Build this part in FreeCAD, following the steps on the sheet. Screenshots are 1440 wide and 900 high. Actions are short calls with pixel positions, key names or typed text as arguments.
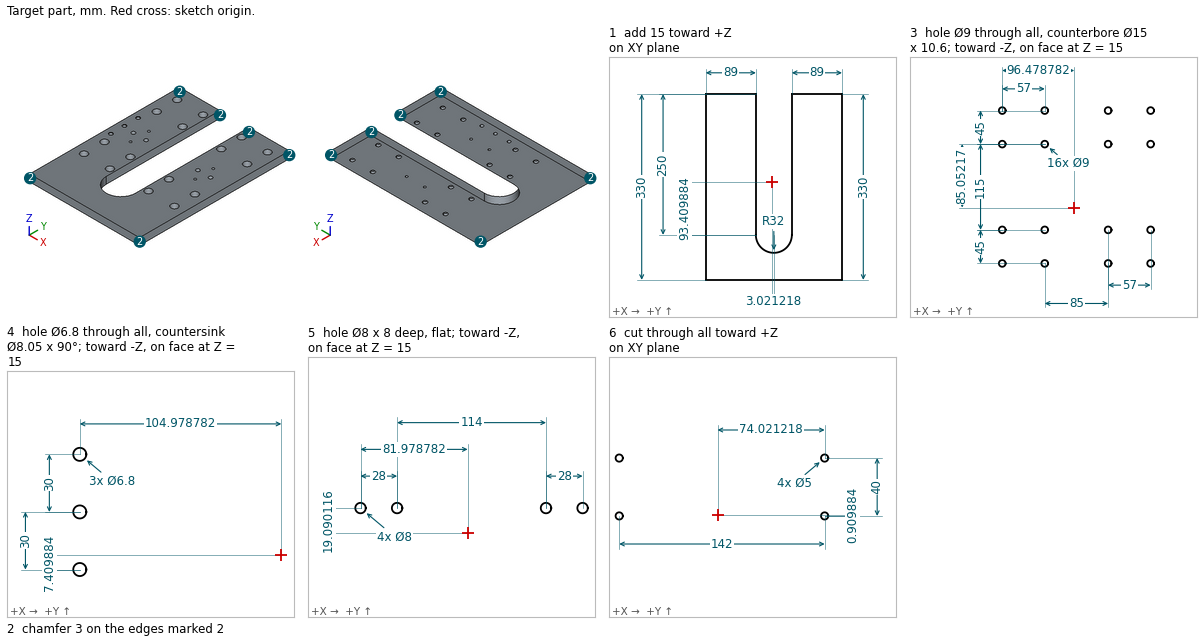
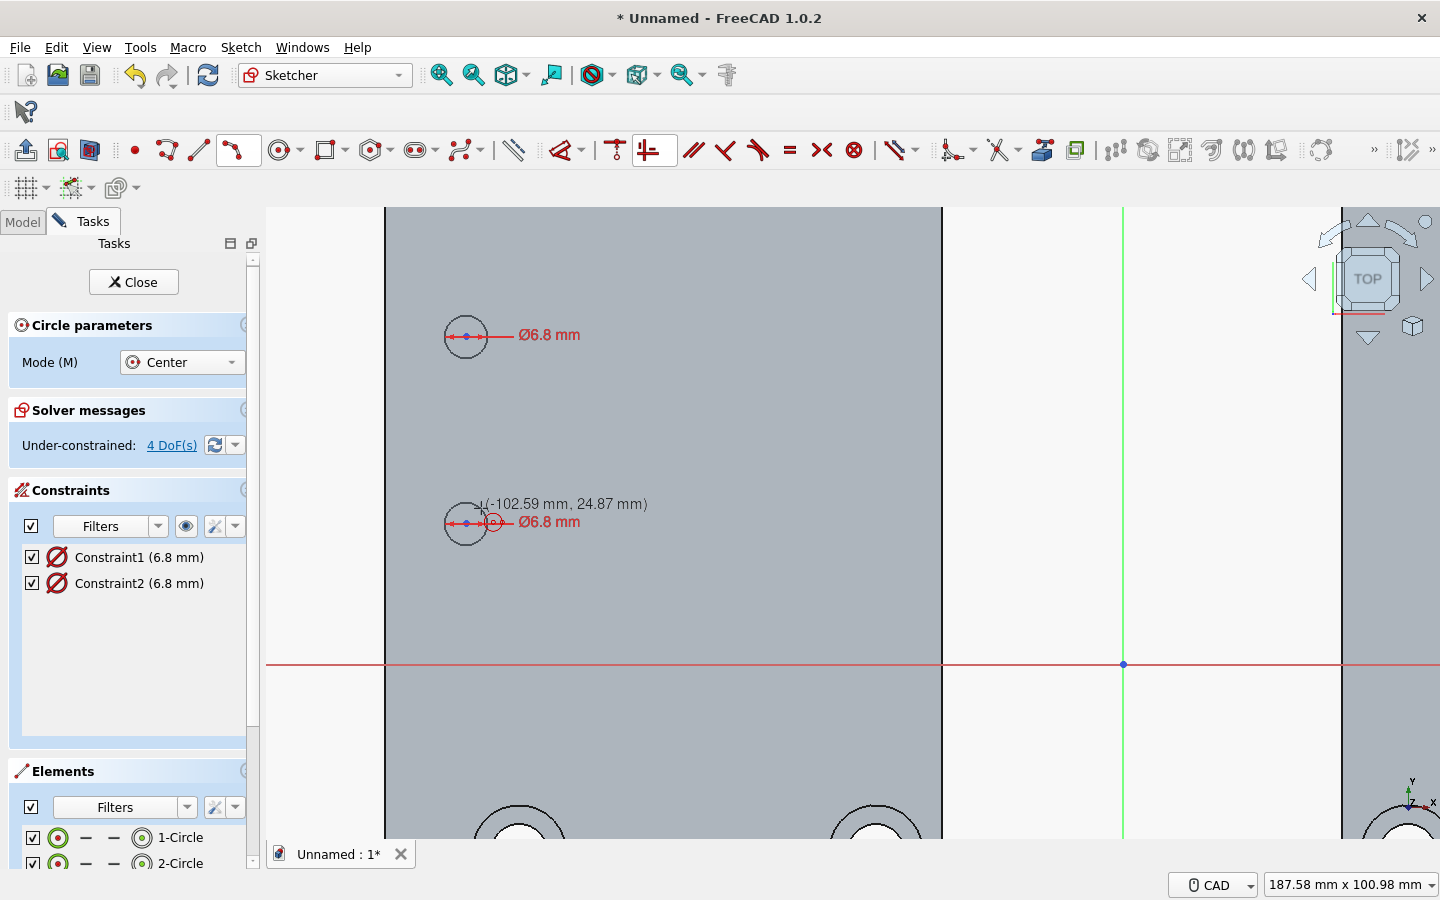
click(466, 711)
move(481, 696)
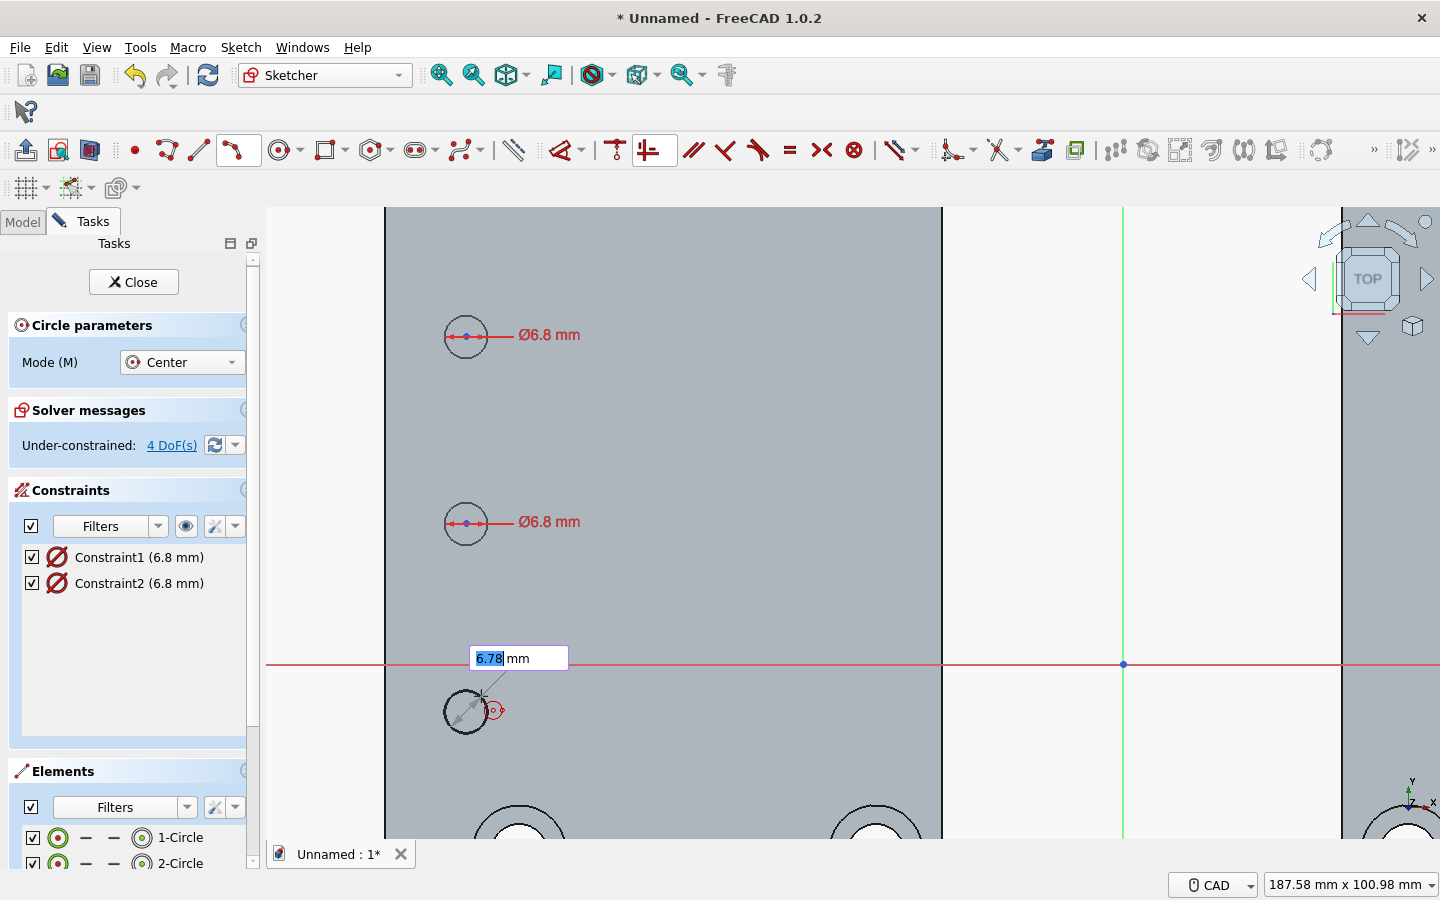
text(6.8)
key(Return)
key(Escape)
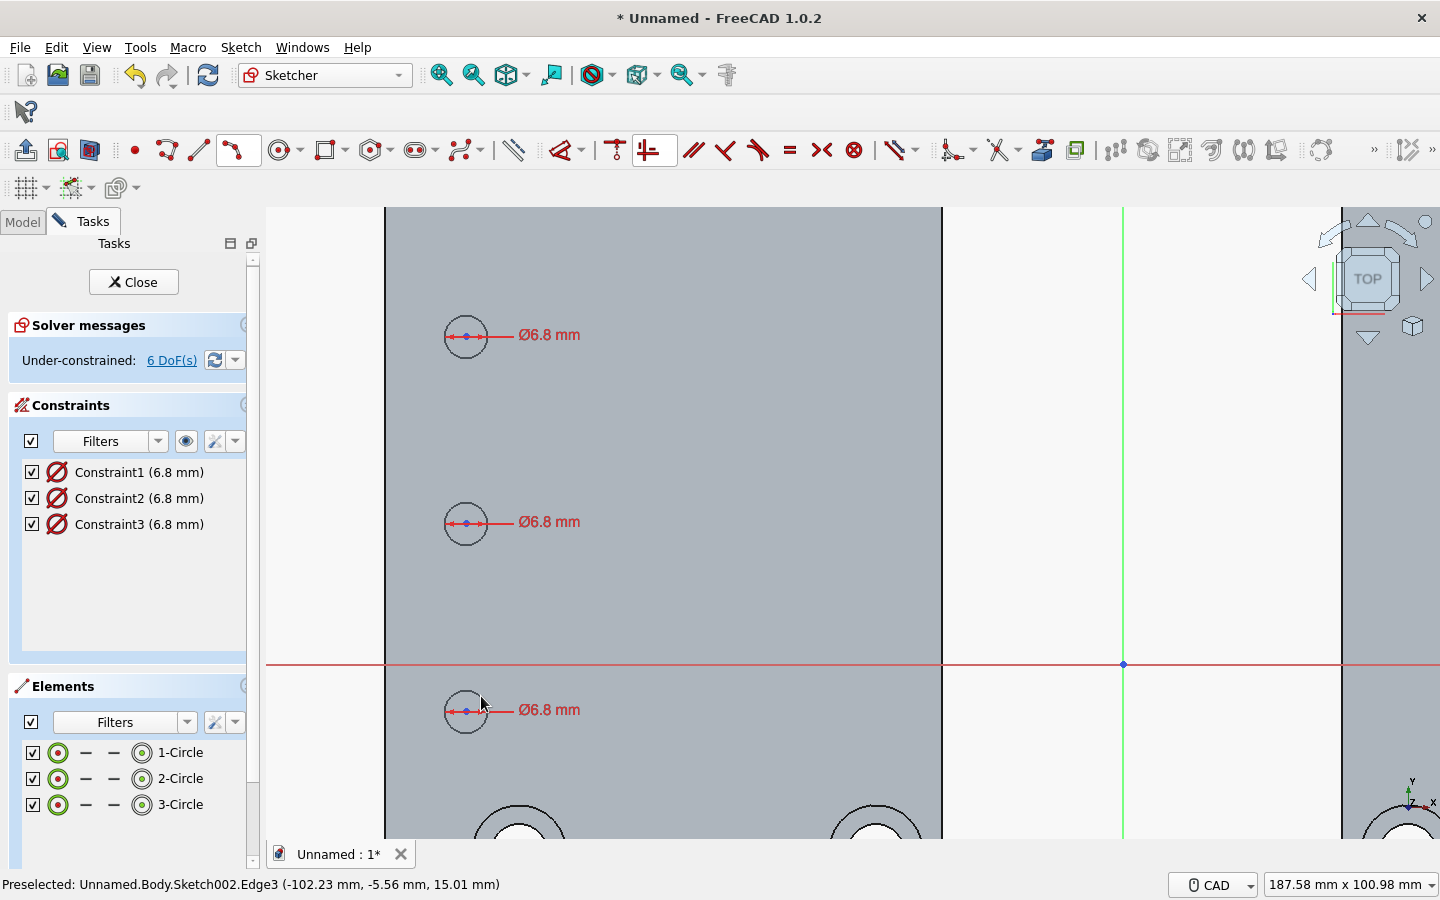
click(466, 337)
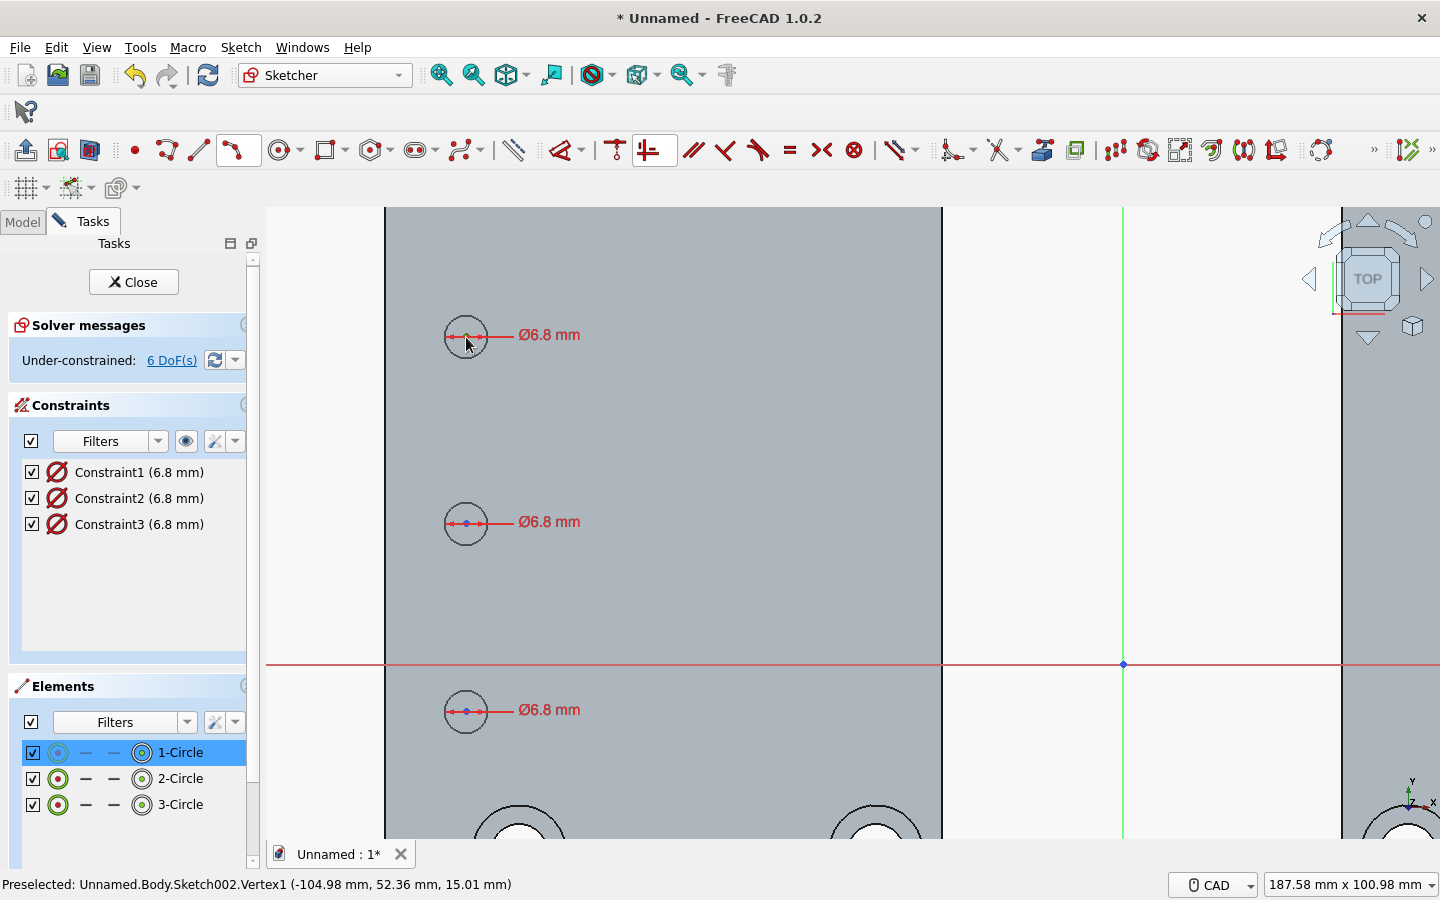
click(466, 524)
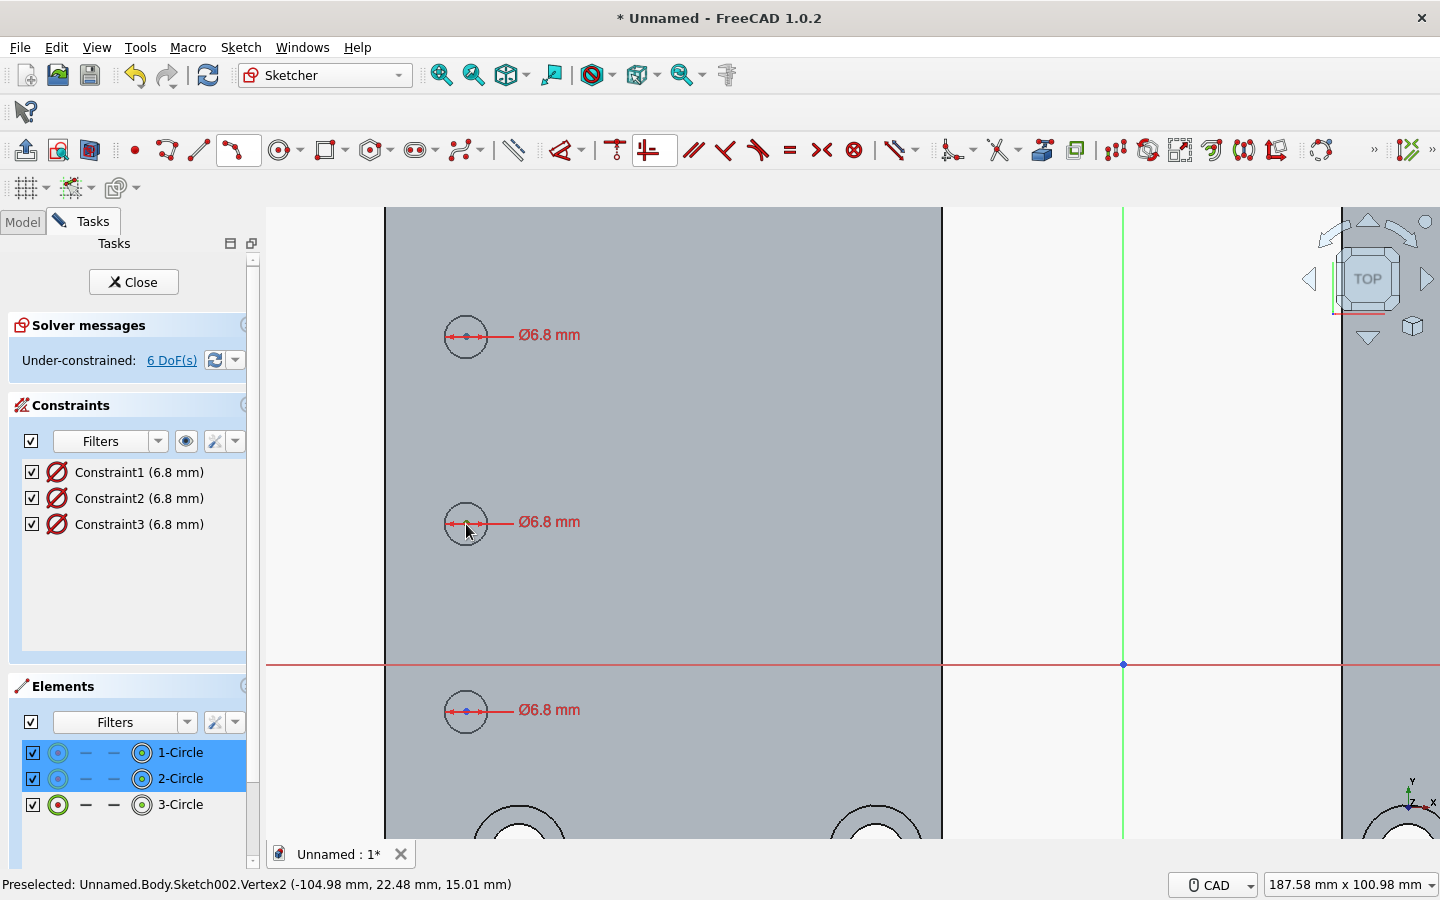
key(v)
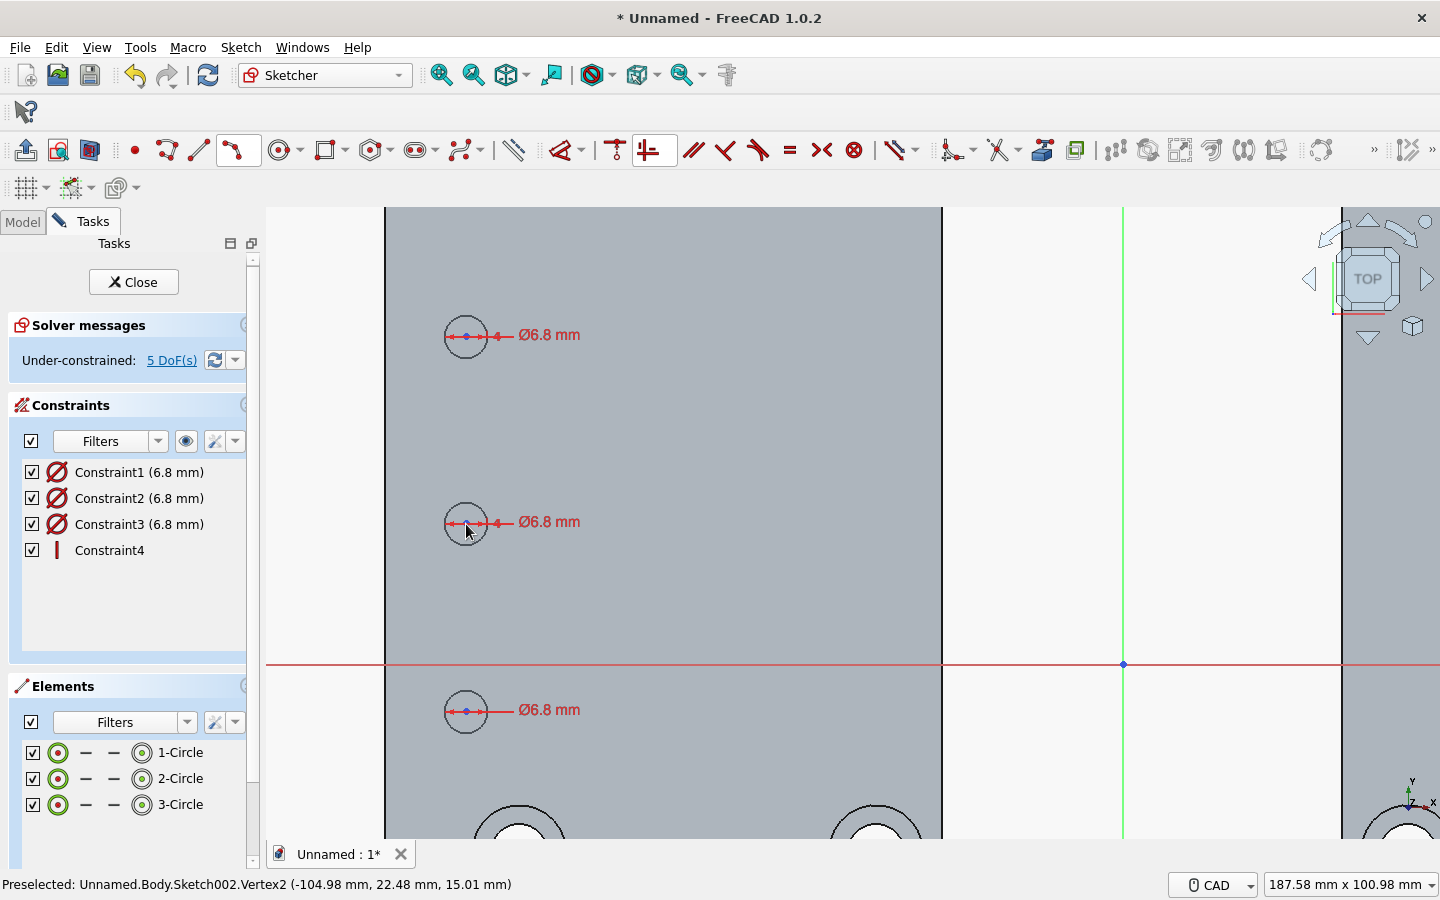
click(466, 524)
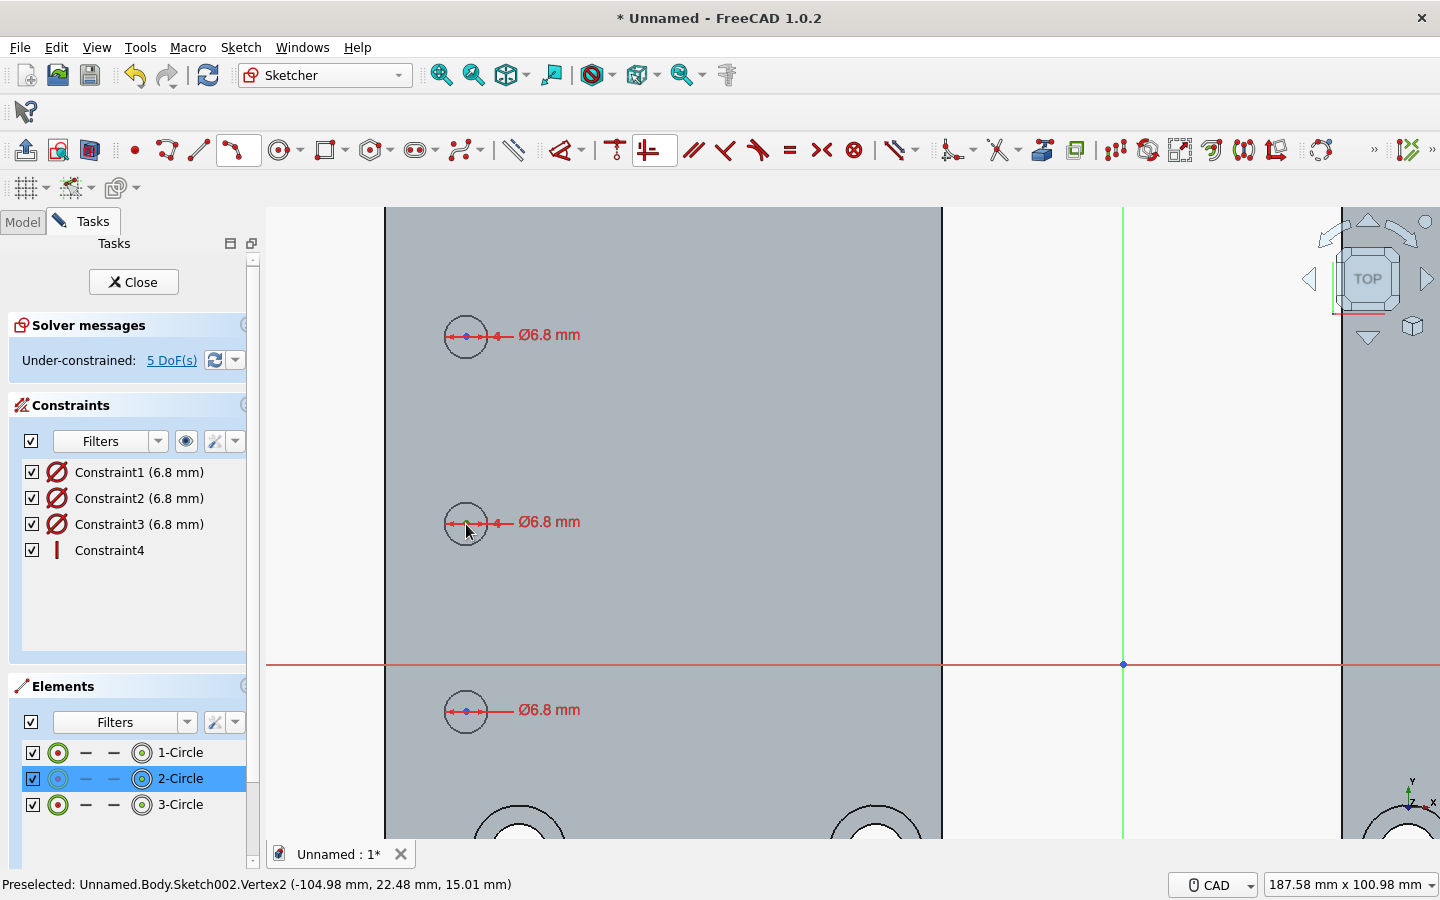
click(466, 712)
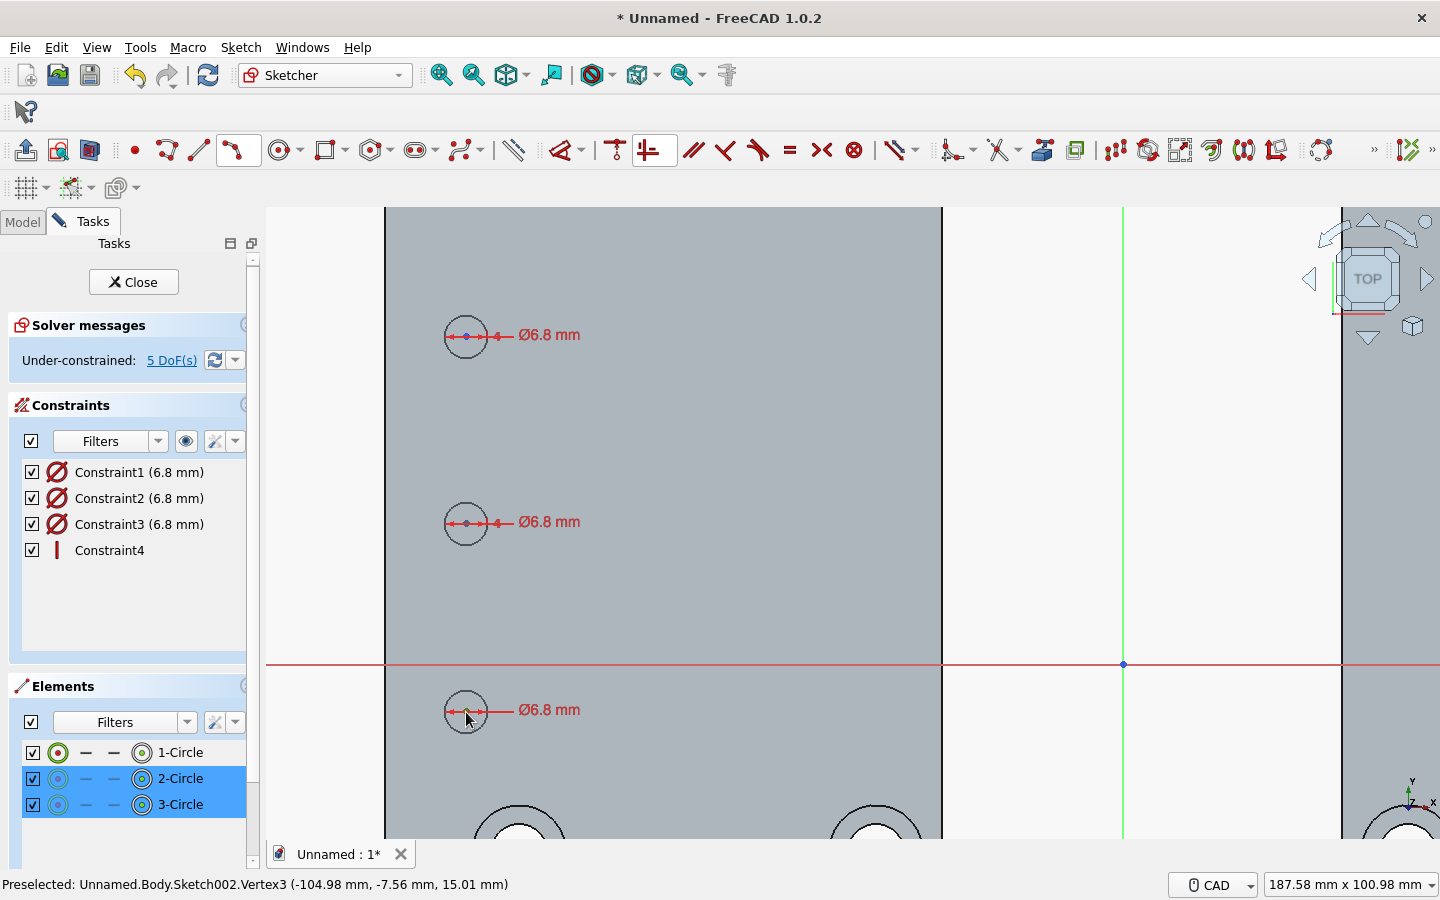
click(672, 150)